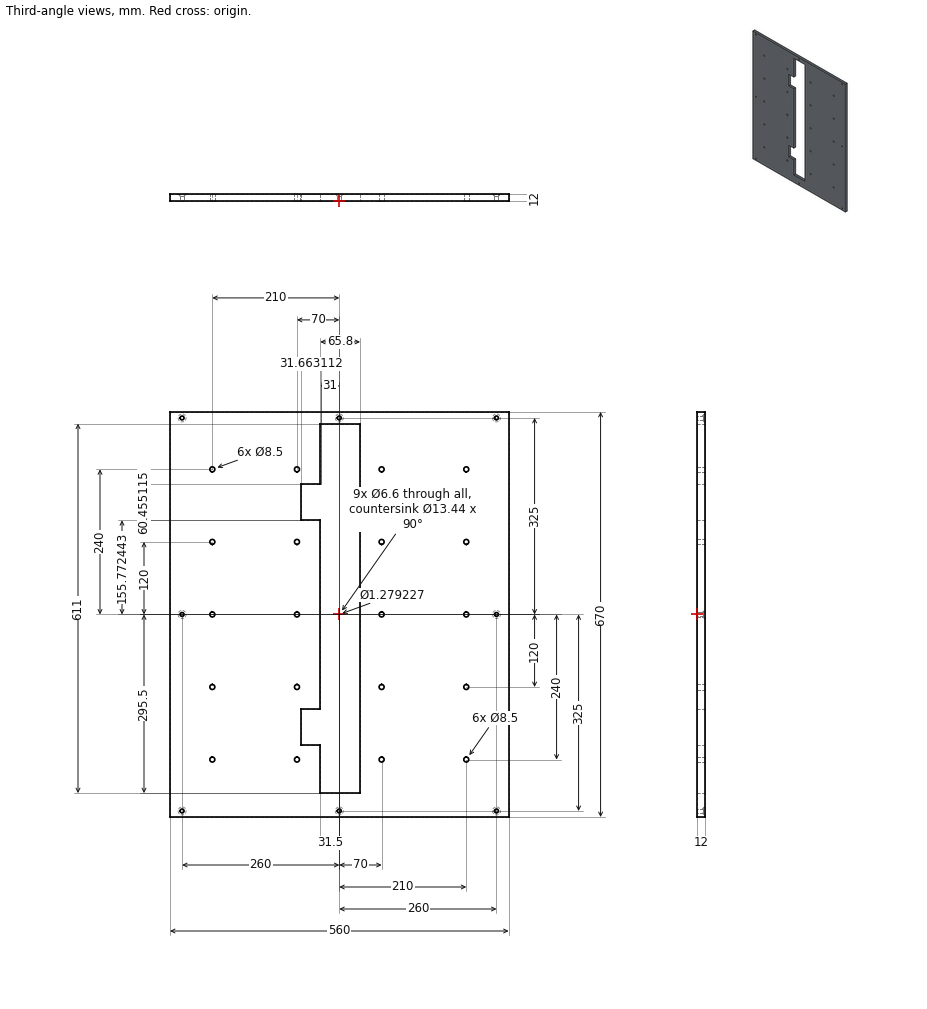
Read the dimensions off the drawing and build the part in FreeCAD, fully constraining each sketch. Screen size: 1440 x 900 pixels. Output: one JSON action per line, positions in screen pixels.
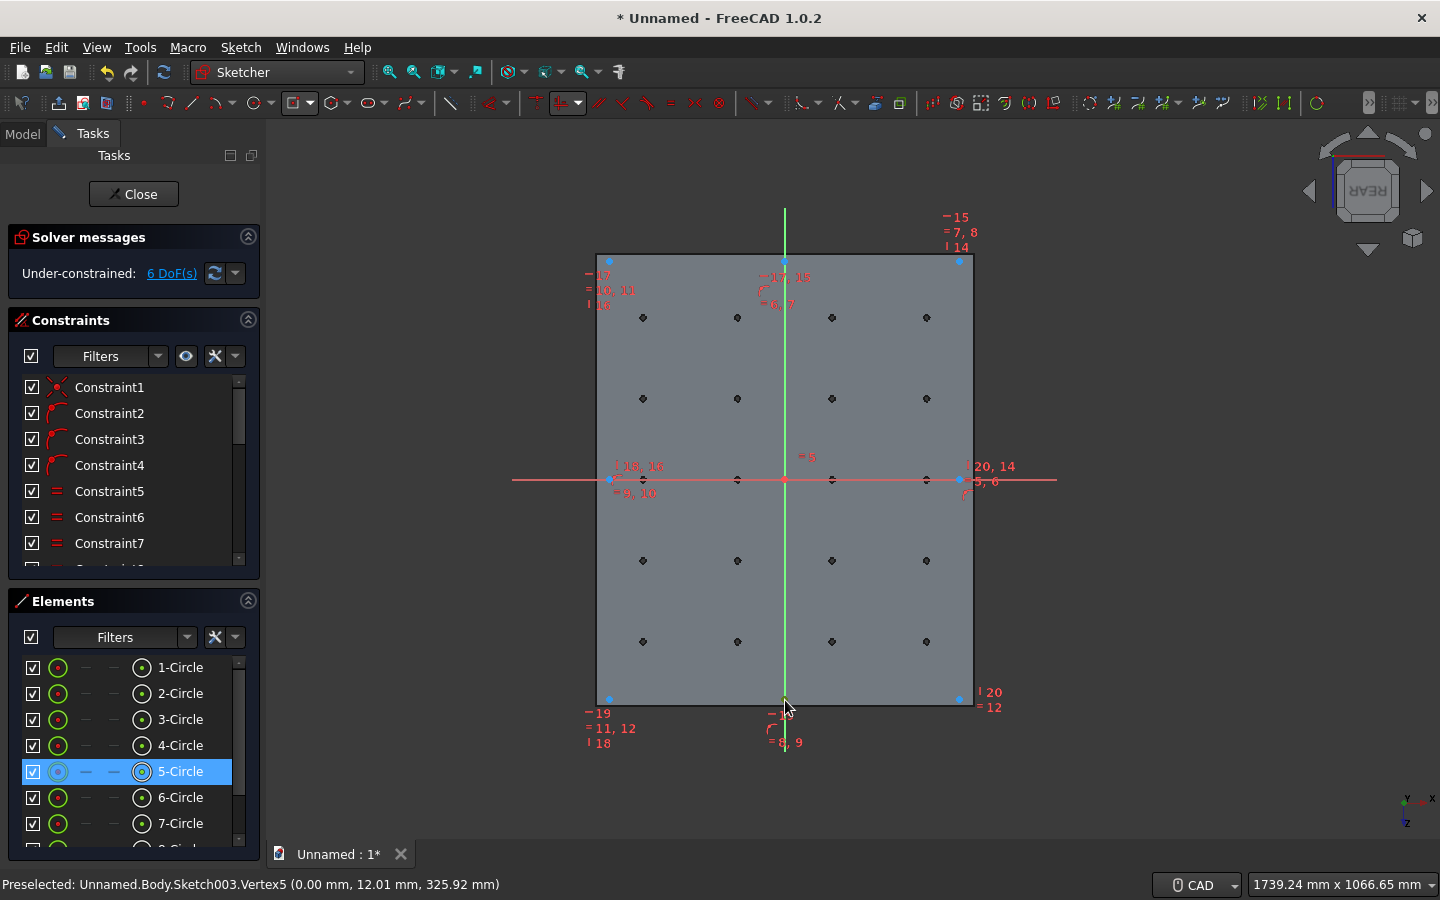
{"action": "left_click", "coordinate": [960, 700]}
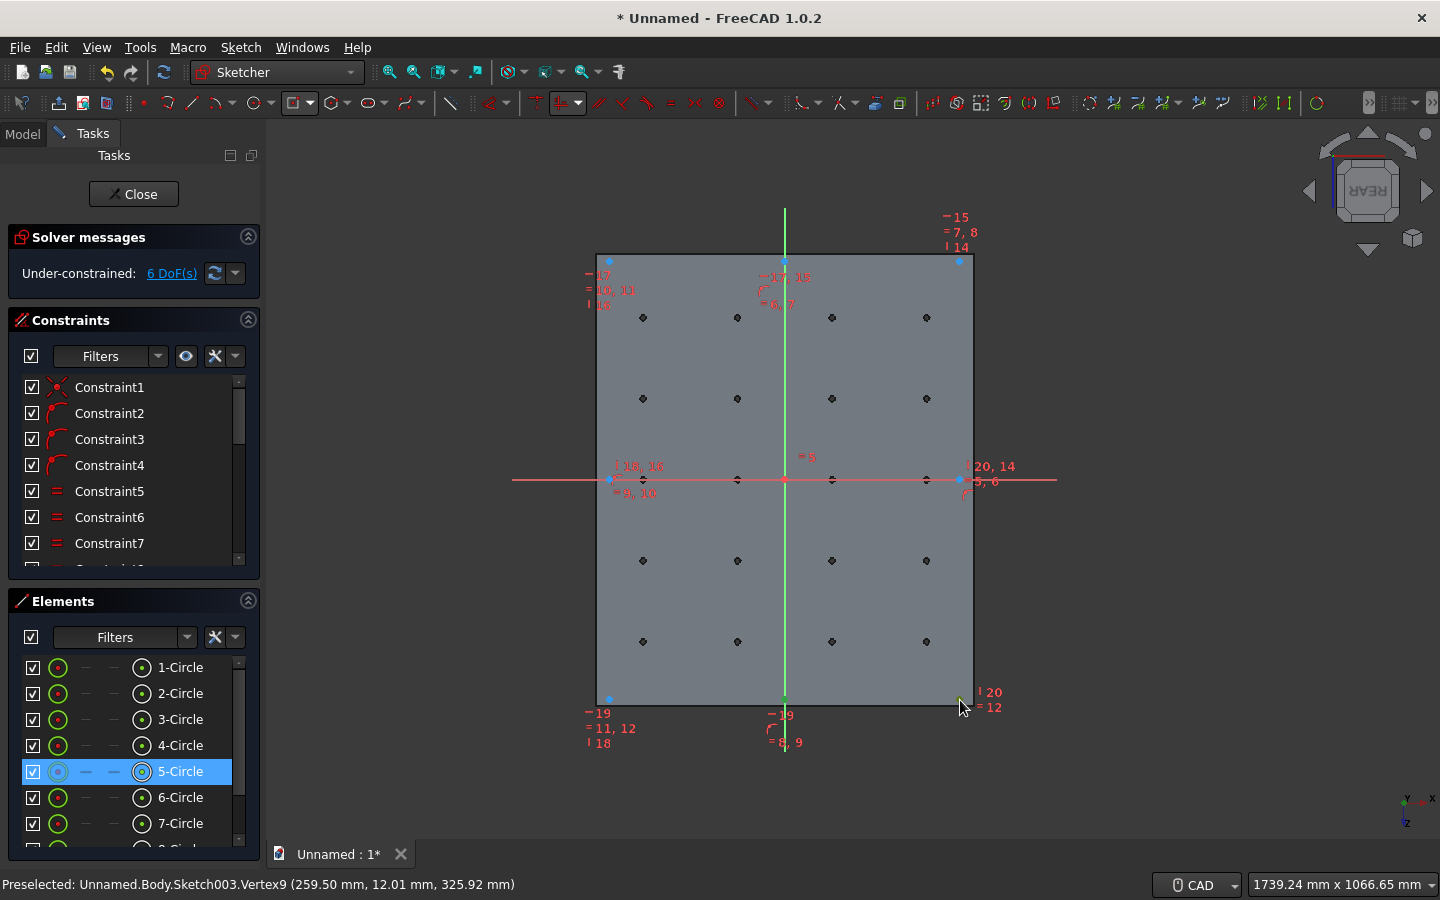
{"action": "key", "text": "h"}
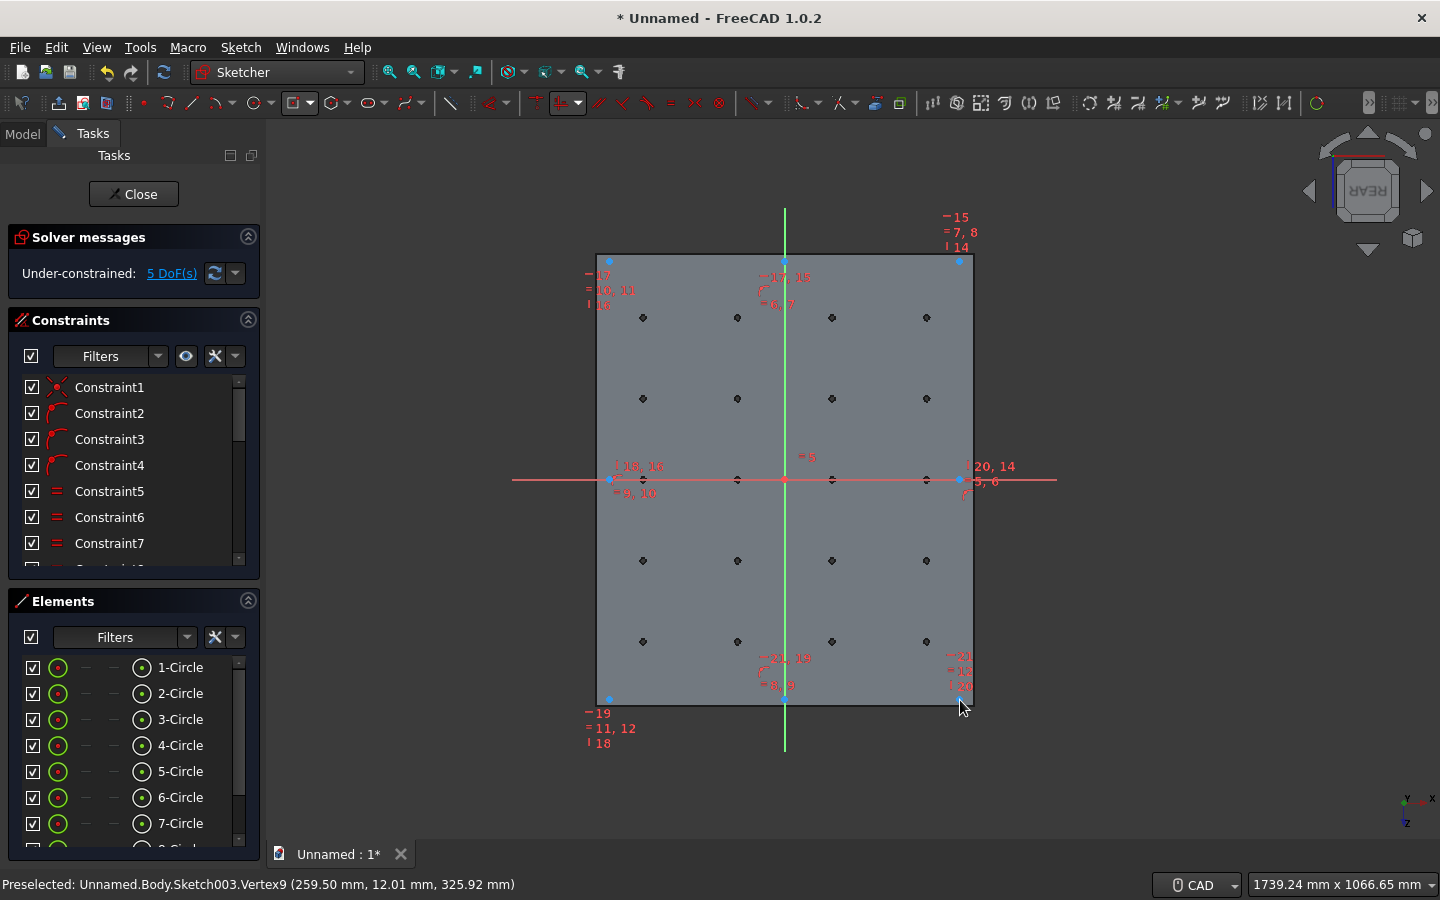
{"action": "left_click", "coordinate": [490, 104]}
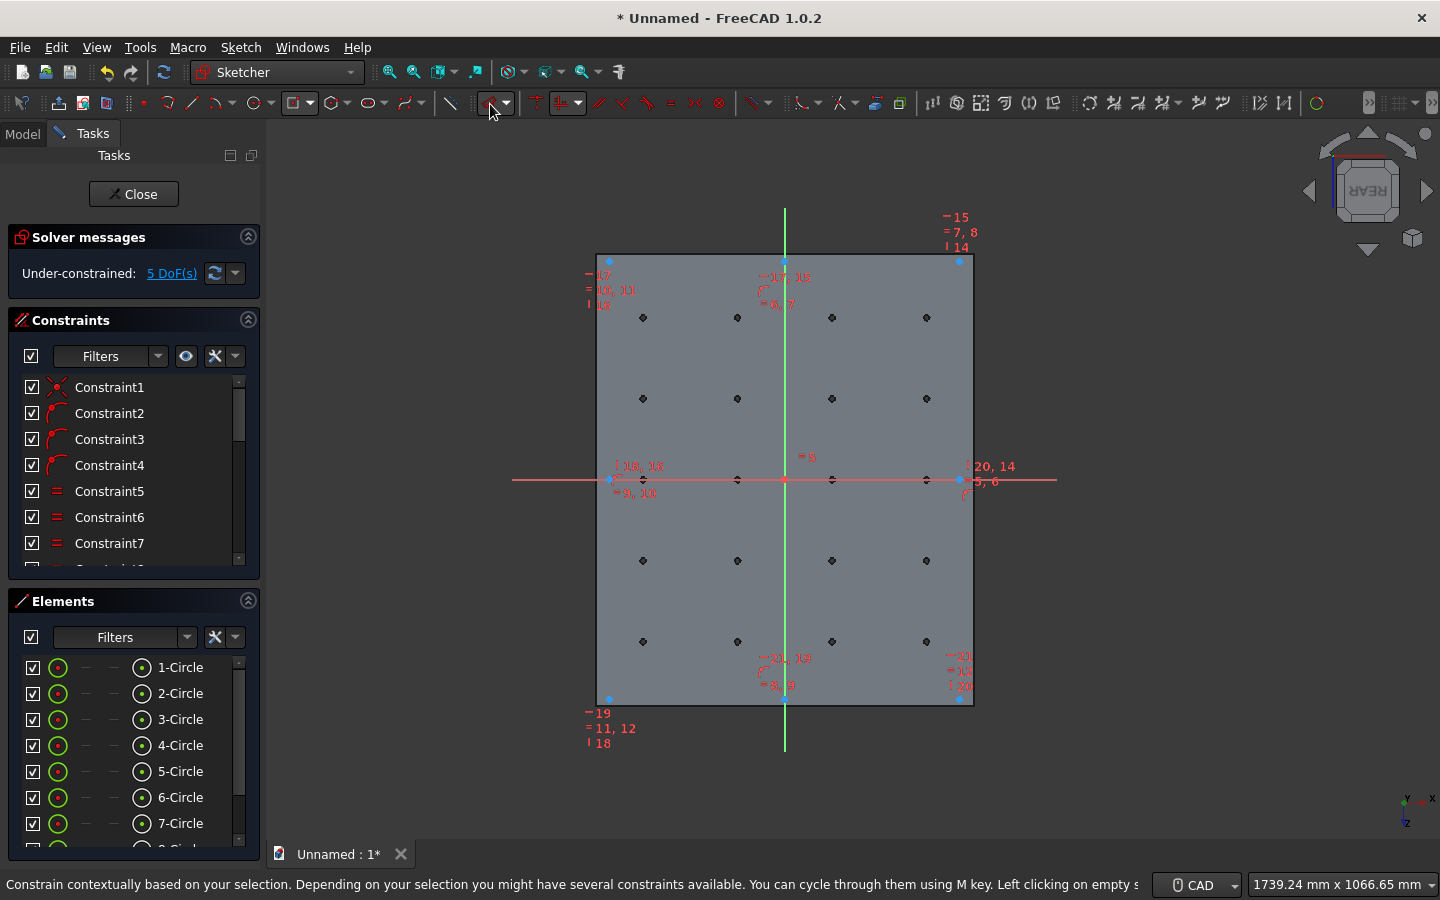
{"action": "scroll", "coordinate": [786, 478], "scroll_direction": "up", "scroll_amount": 11}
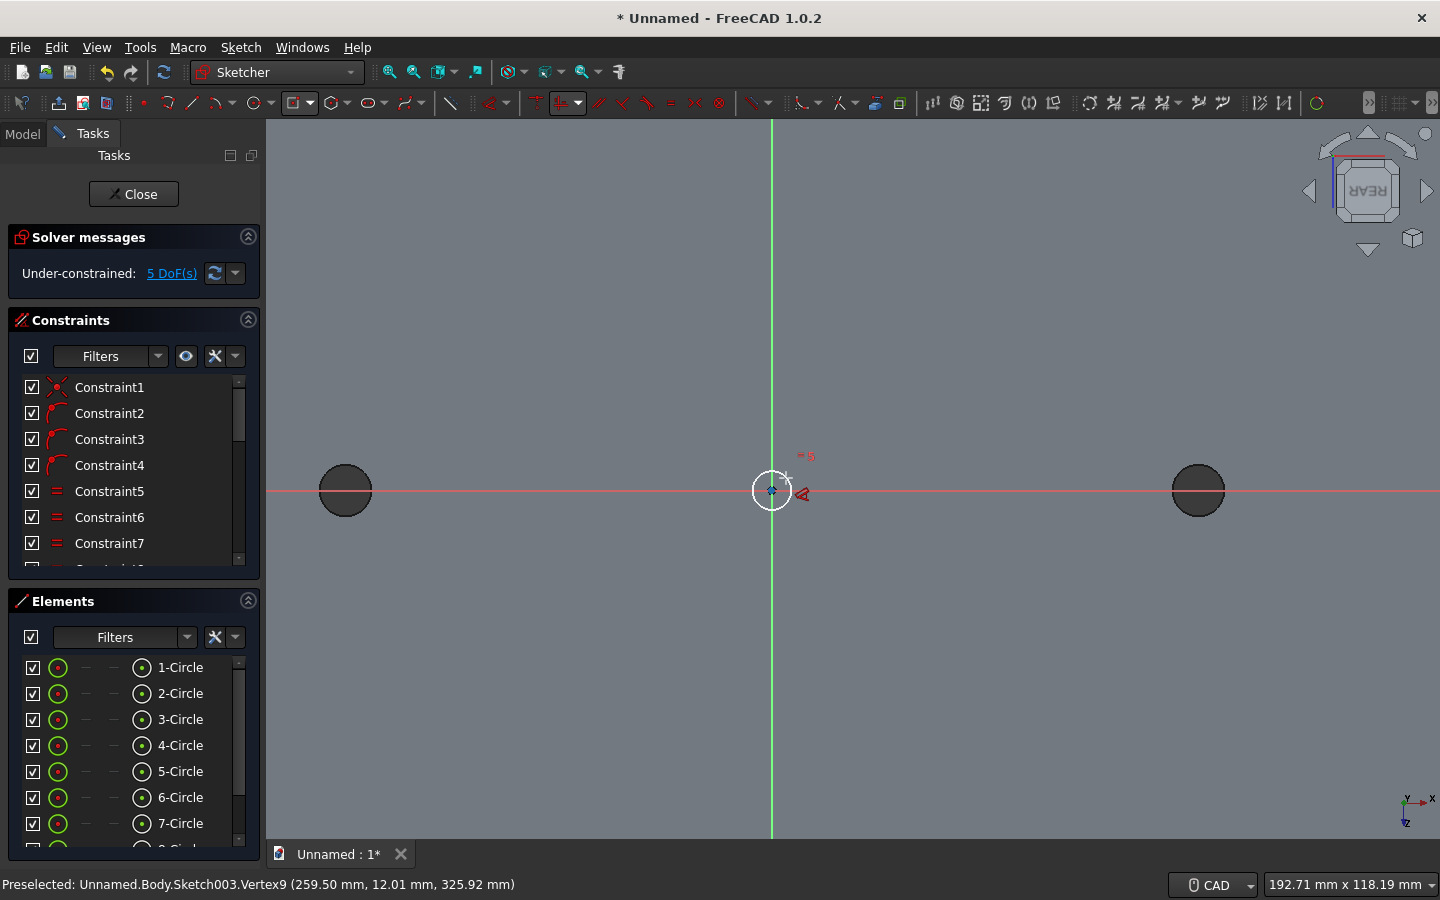
{"action": "left_click", "coordinate": [786, 477]}
{"action": "left_click", "coordinate": [809, 455]}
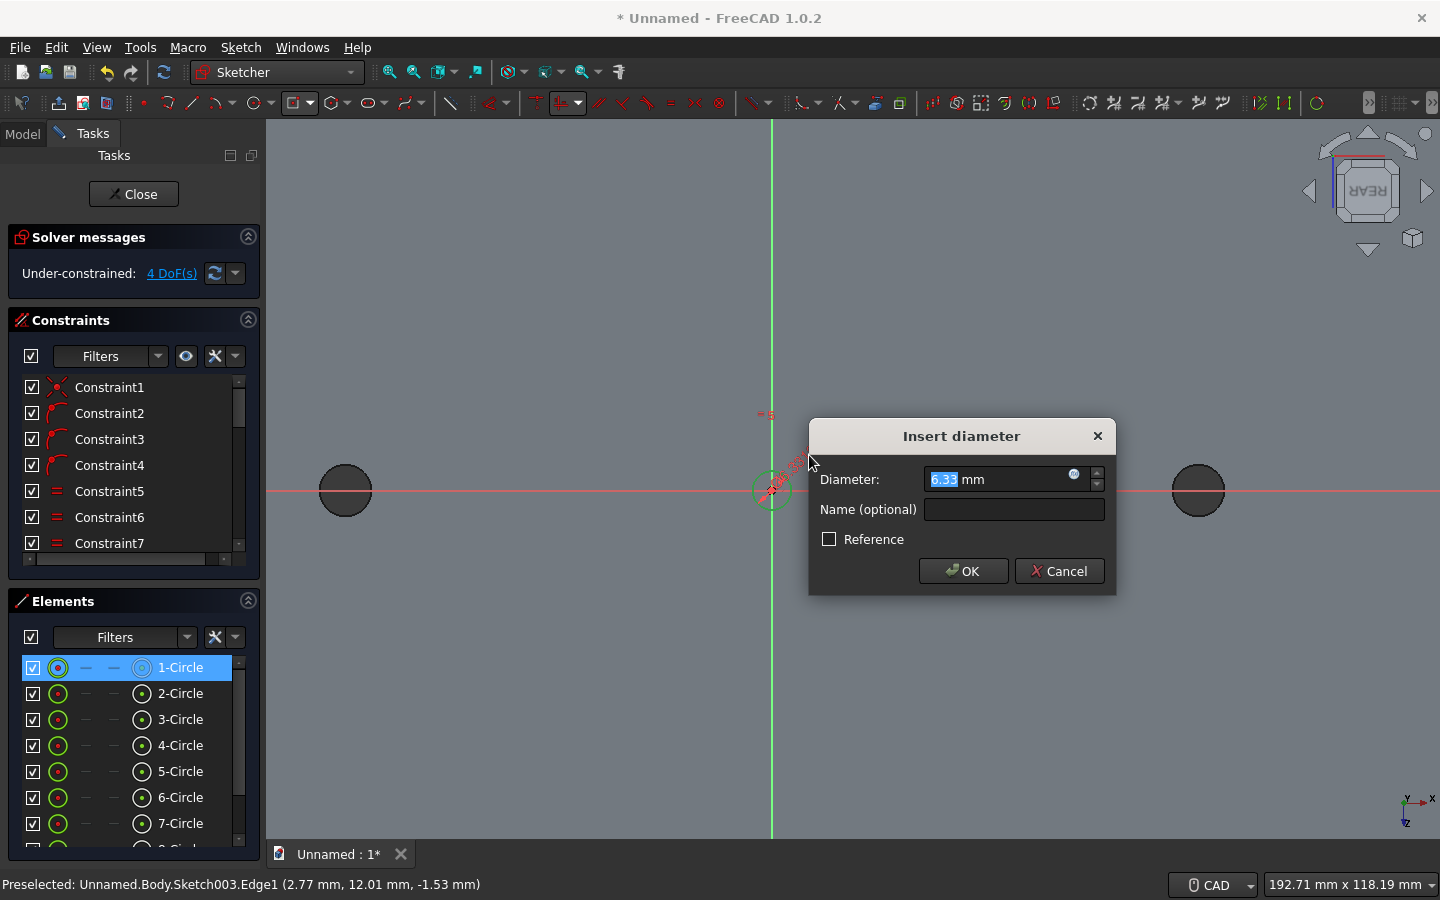
{"action": "type", "text": "6.6"}
{"action": "key", "text": "Return"}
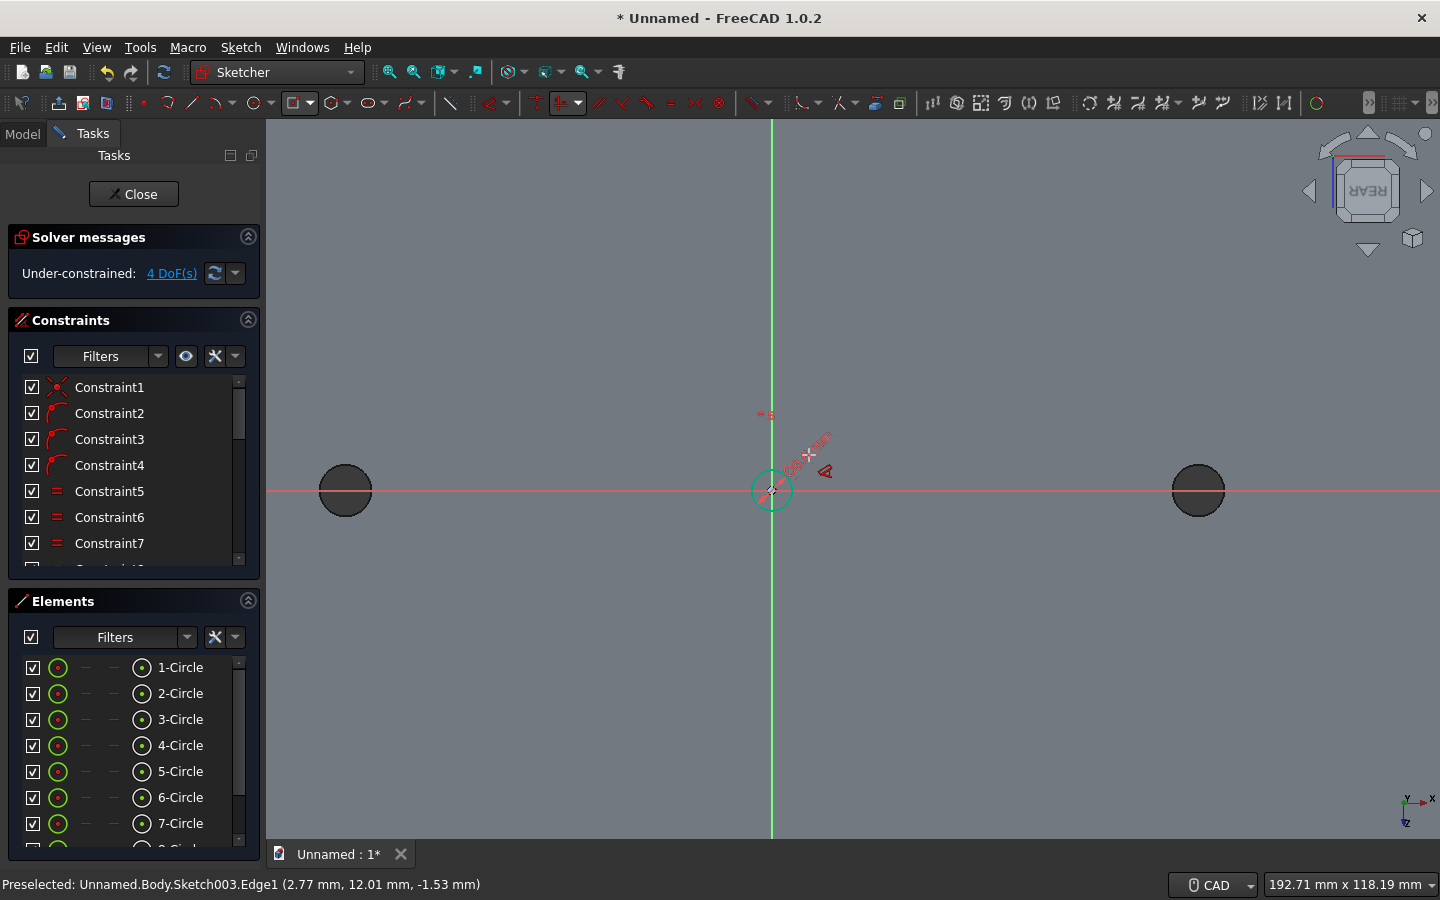
{"action": "scroll", "coordinate": [786, 478], "scroll_direction": "down", "scroll_amount": 11}